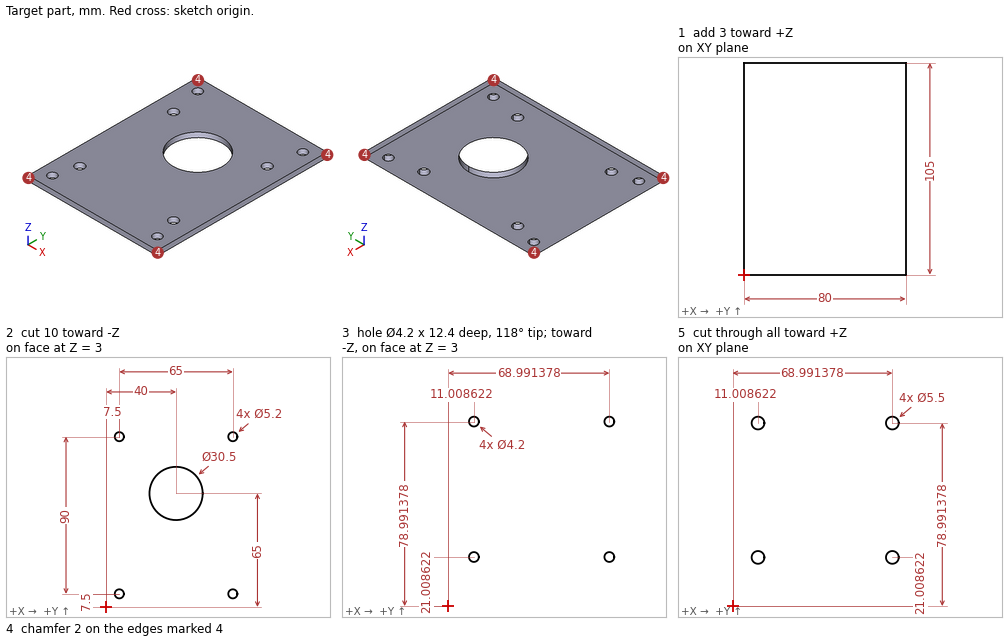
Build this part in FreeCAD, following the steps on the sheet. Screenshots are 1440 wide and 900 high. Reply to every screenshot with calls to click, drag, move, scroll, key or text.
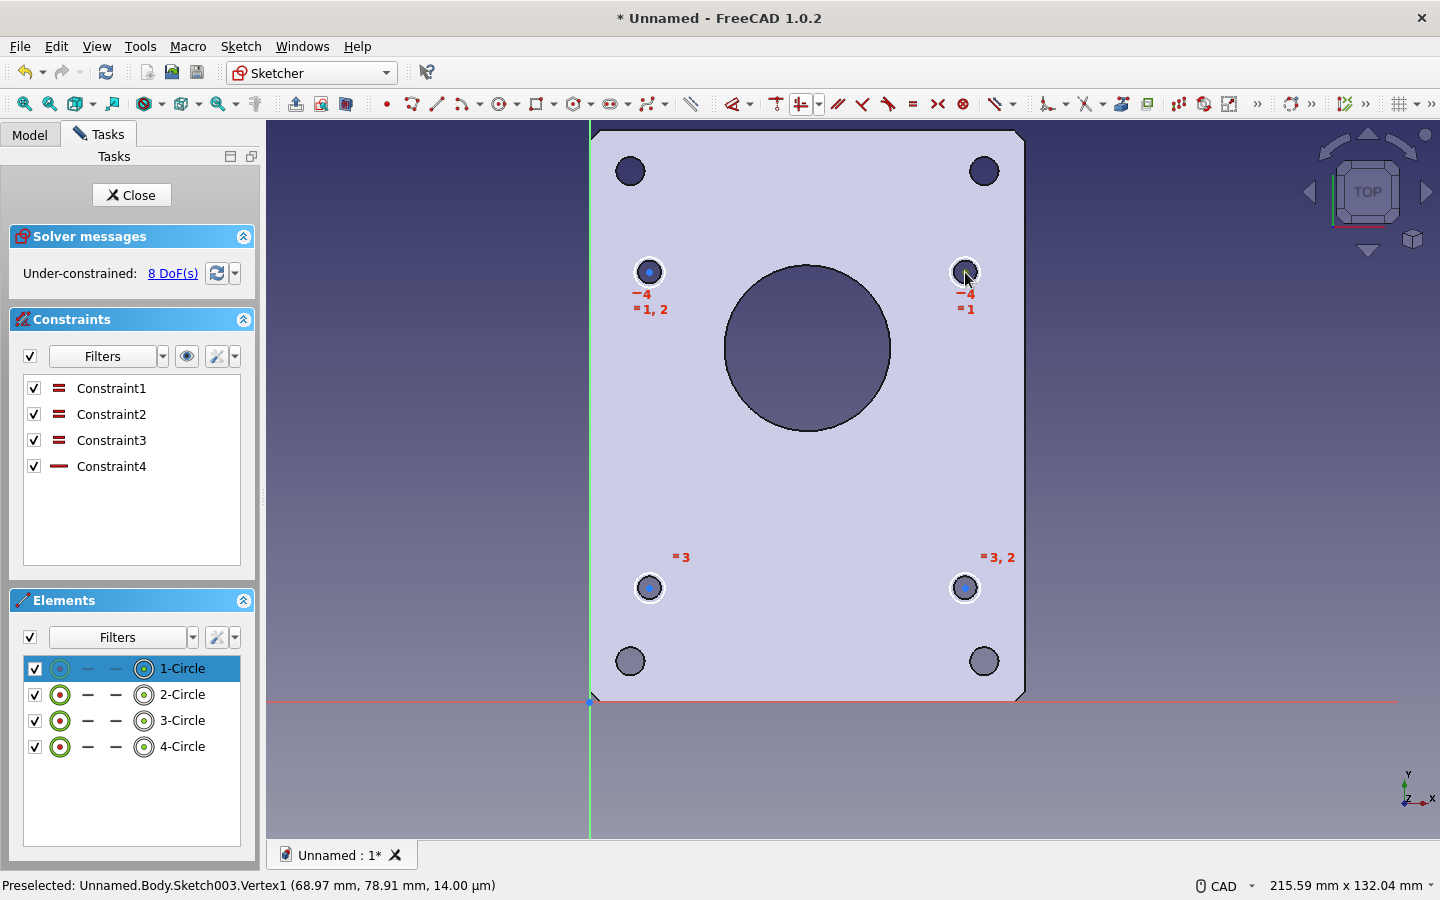
click(965, 588)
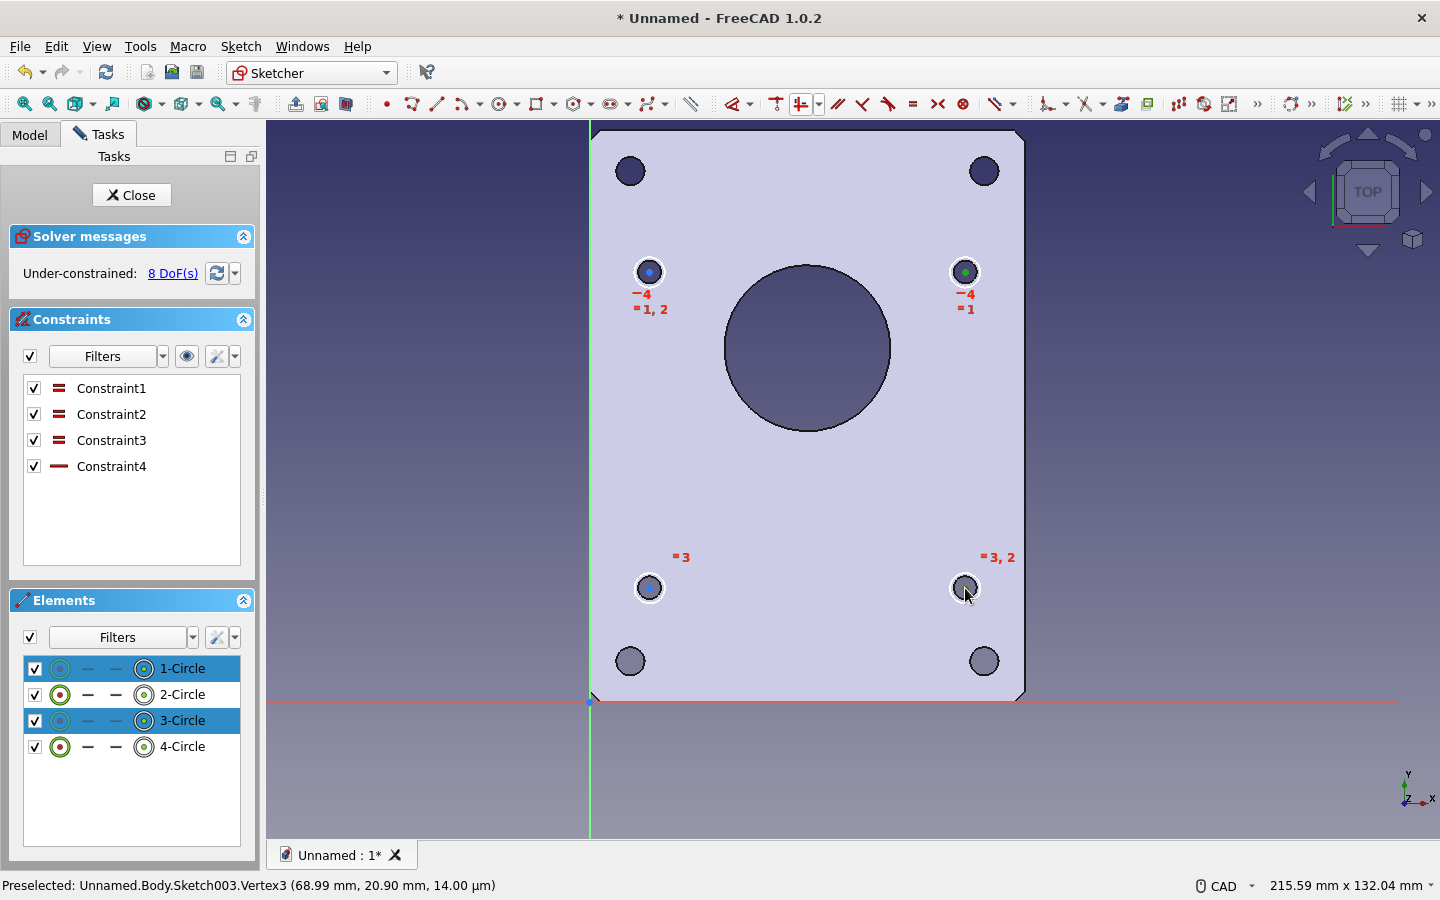
key(v)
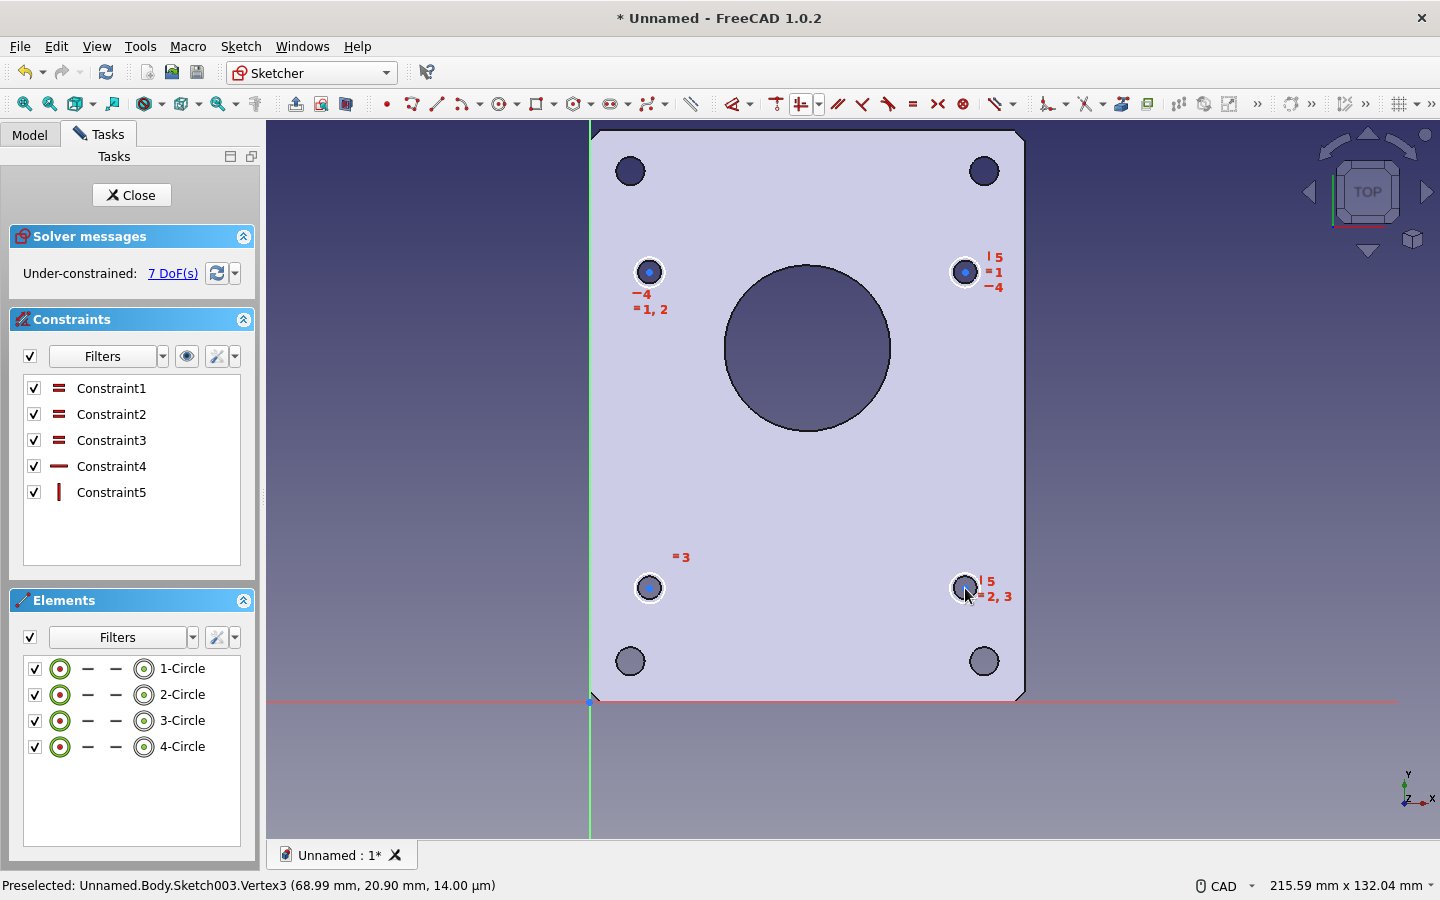
click(650, 272)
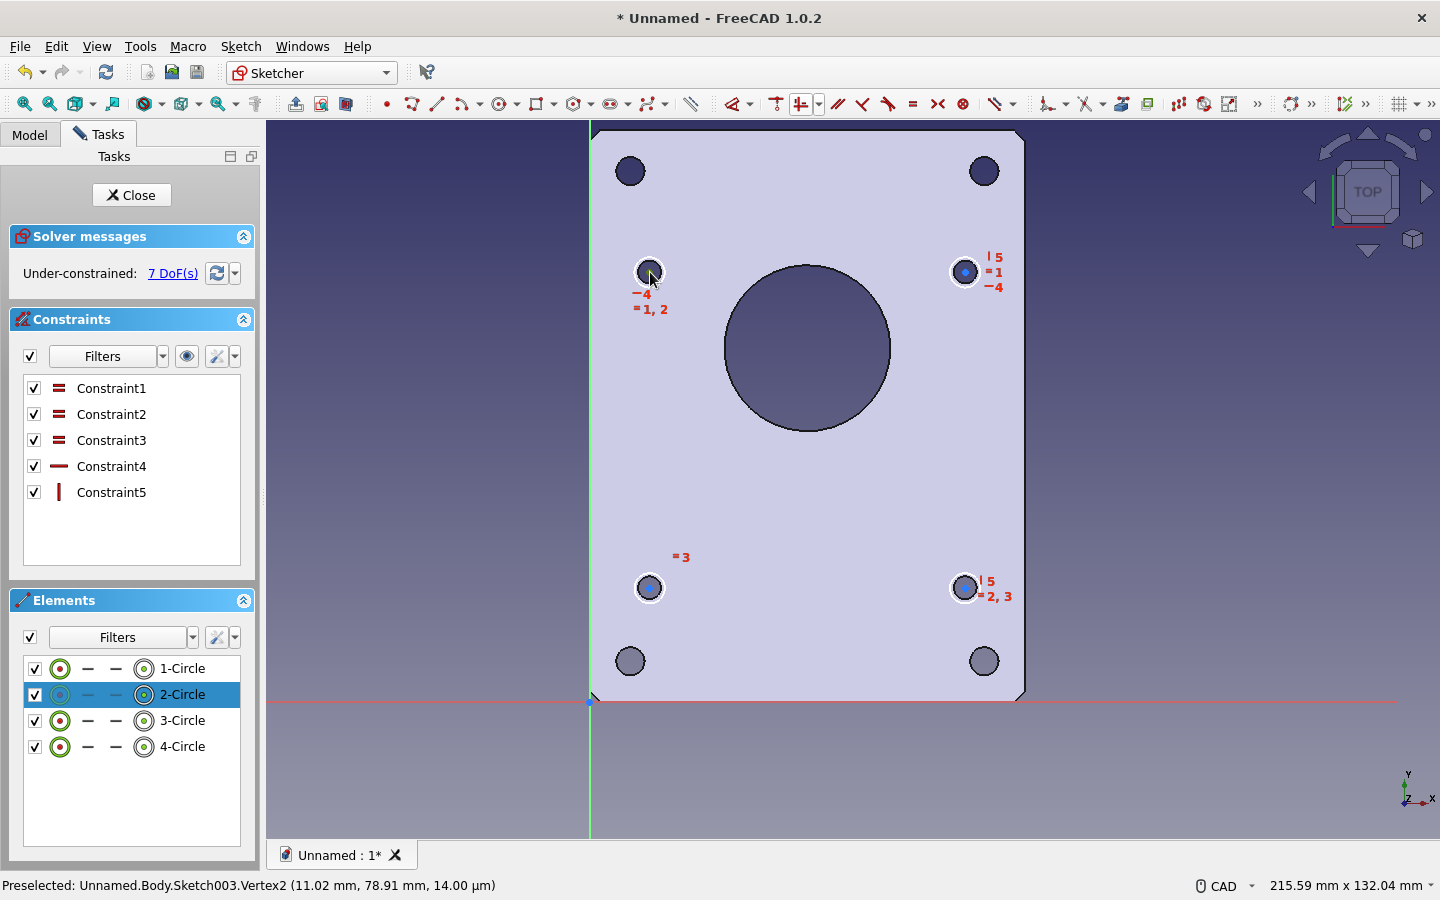
click(650, 588)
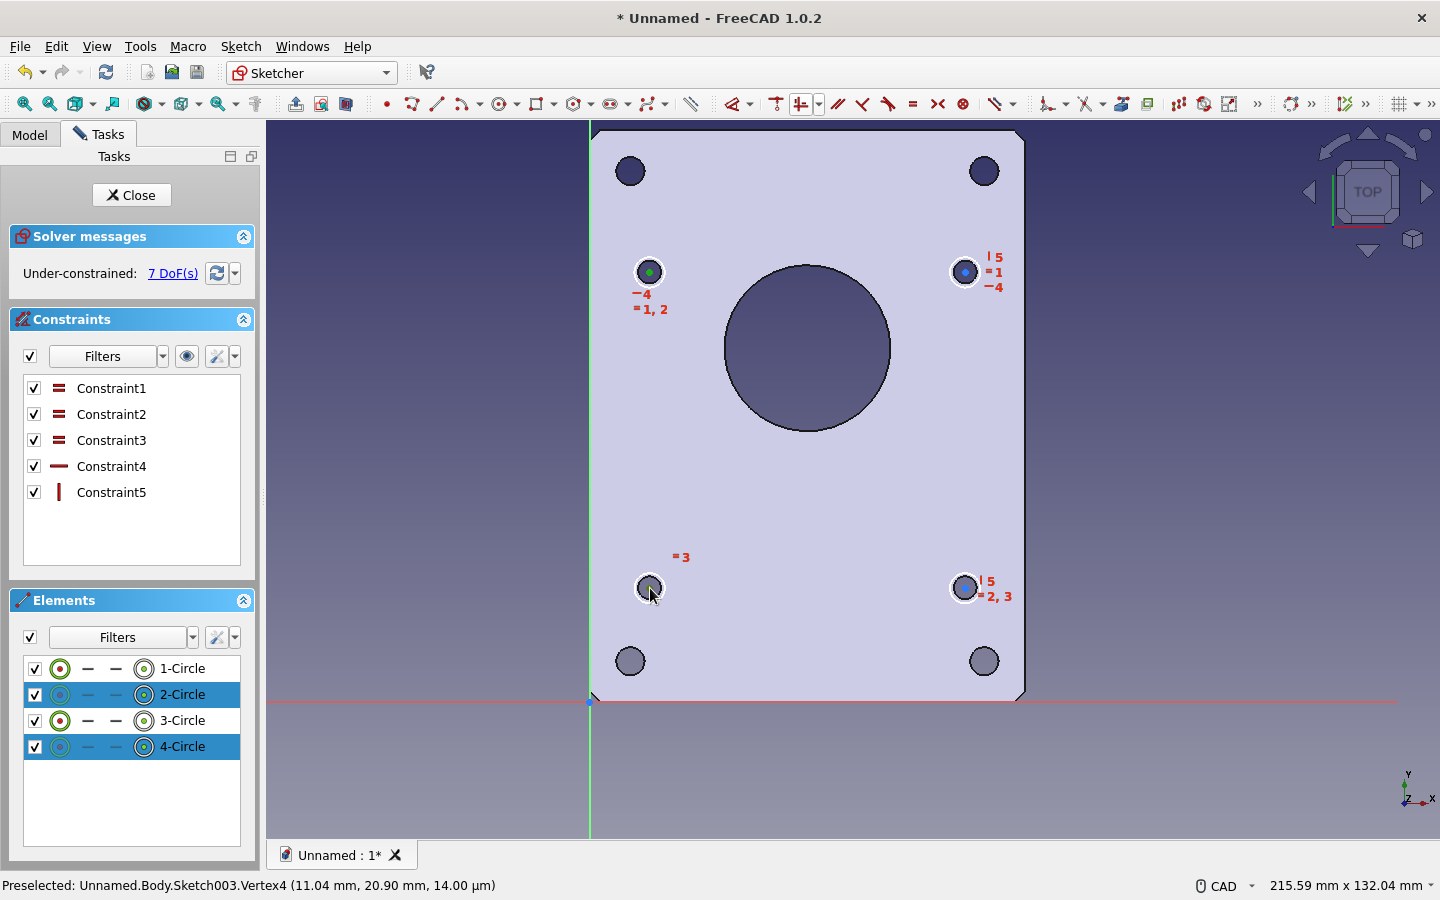
click(818, 104)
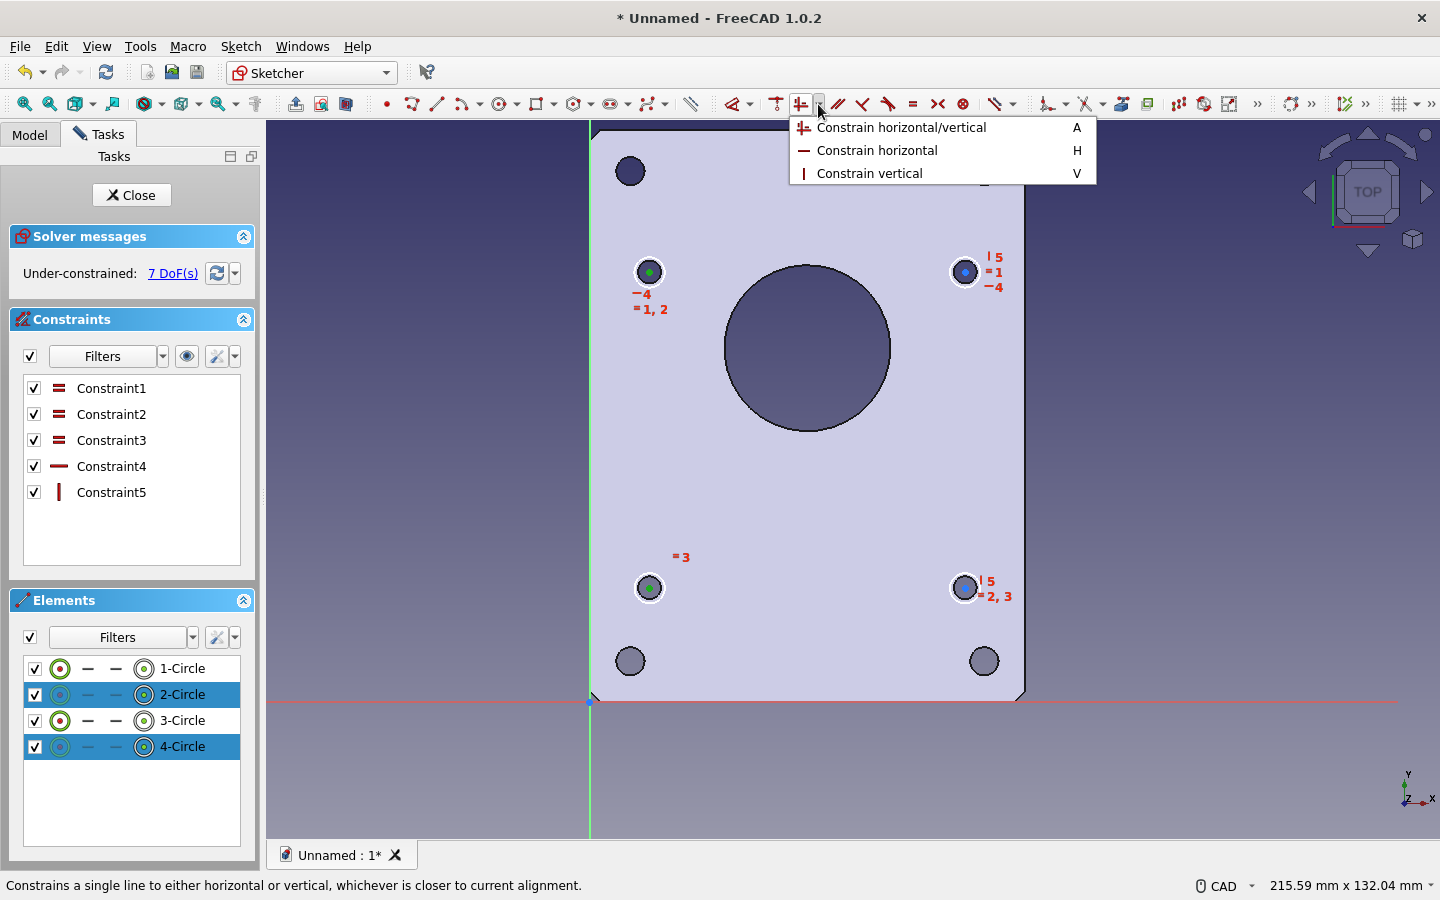
click(943, 174)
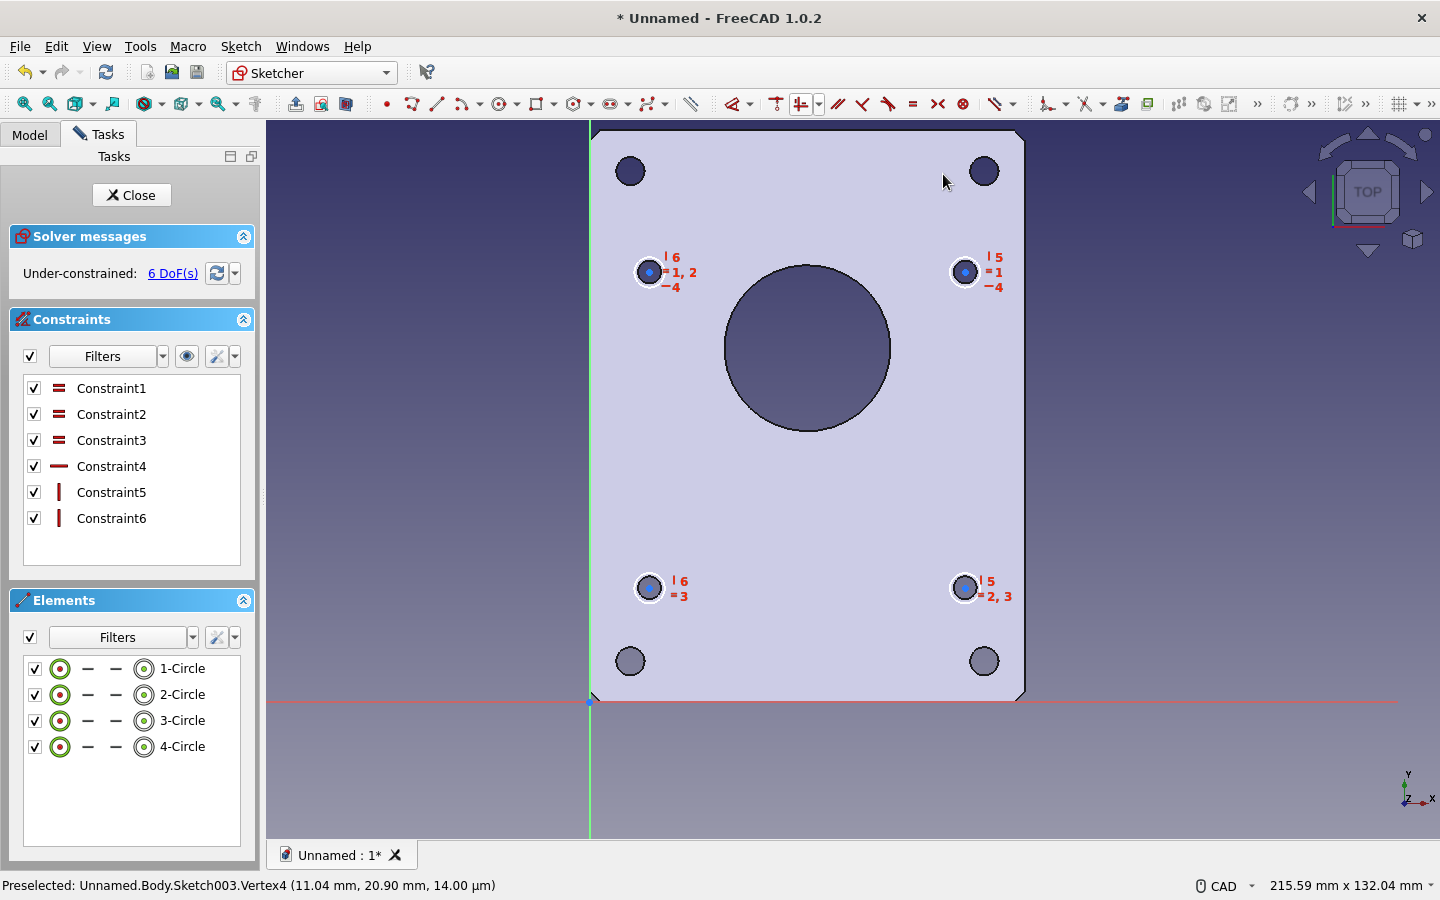
click(965, 588)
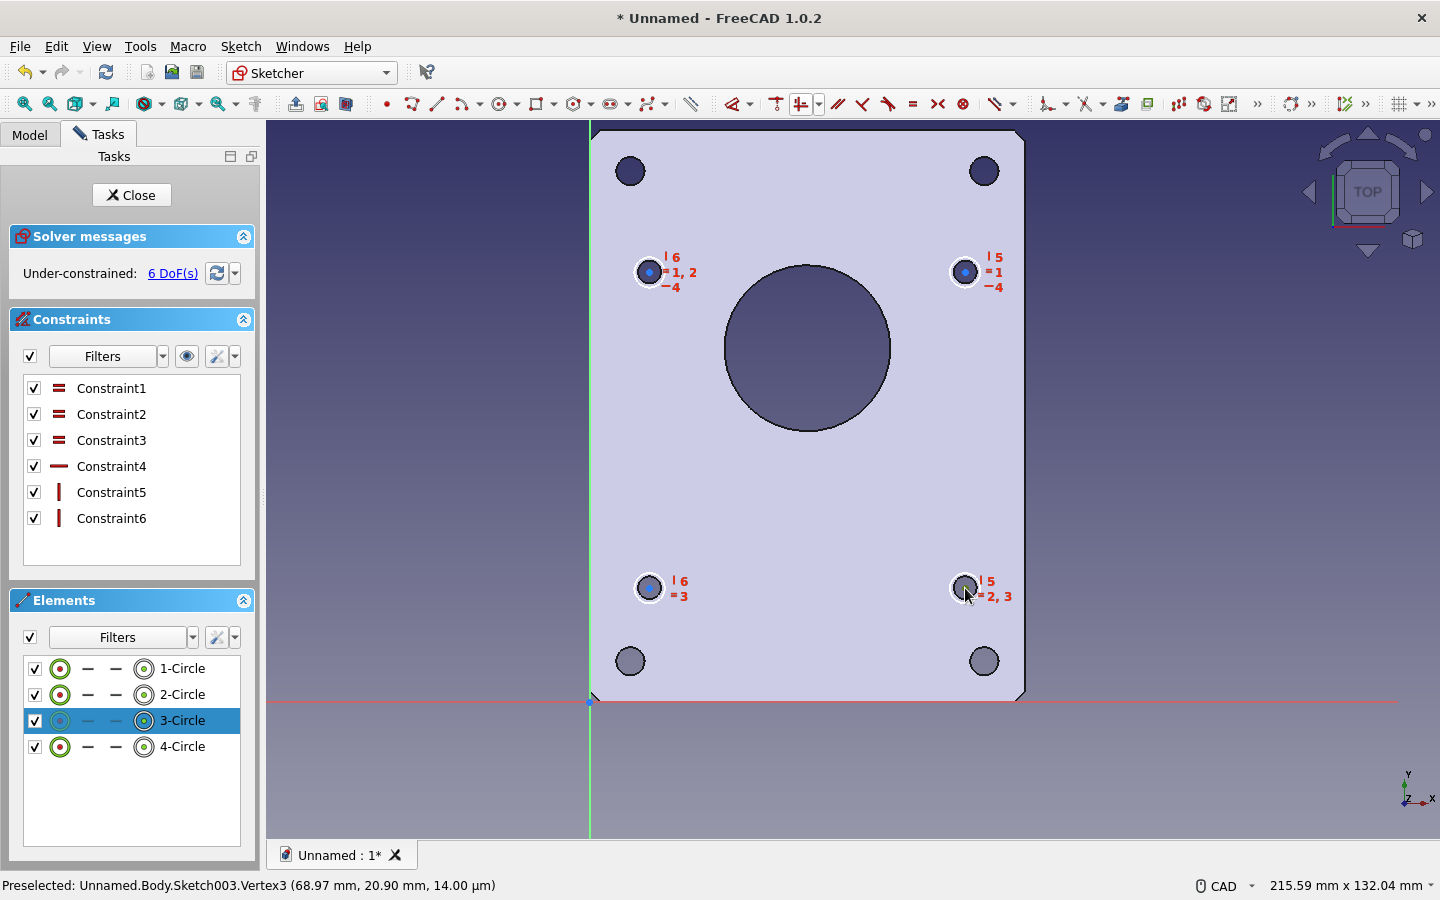
click(650, 588)